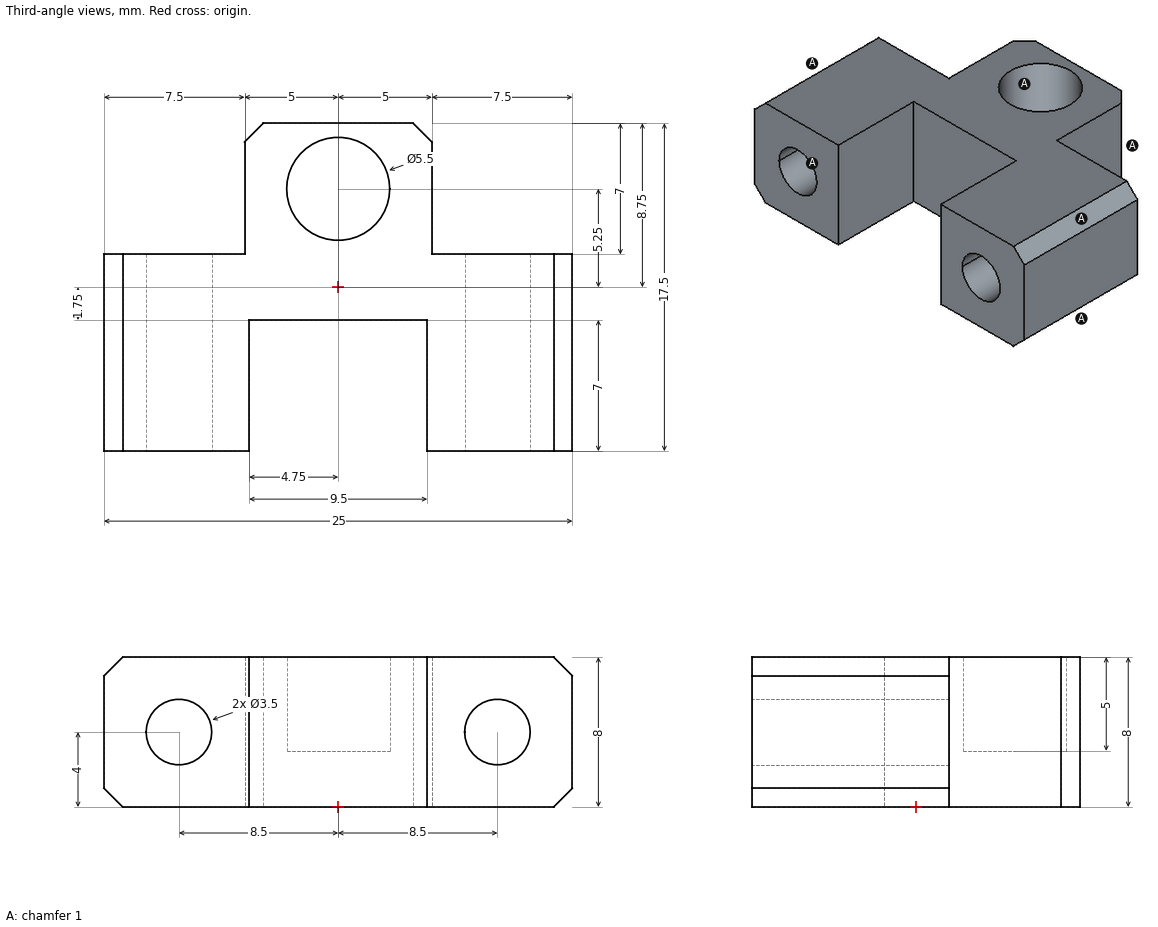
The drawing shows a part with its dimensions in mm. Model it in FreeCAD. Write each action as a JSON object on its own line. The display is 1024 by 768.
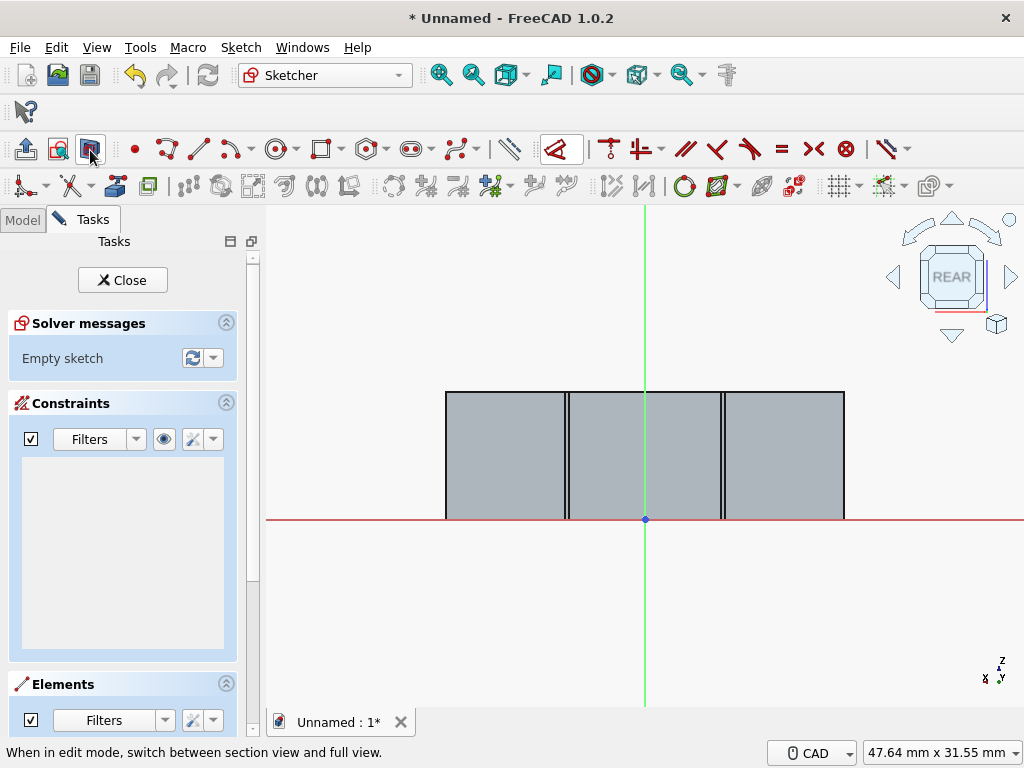
{"action": "key", "text": "g c"}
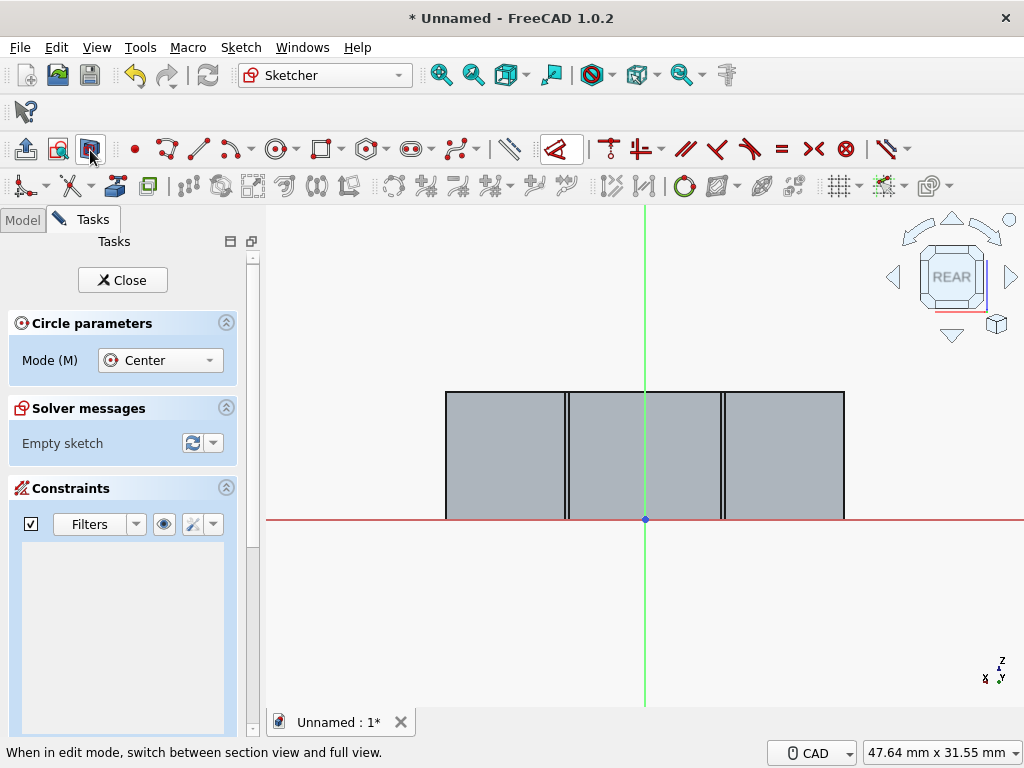
{"action": "left_click", "coordinate": [780, 456]}
{"action": "mouse_move", "coordinate": [800, 436]}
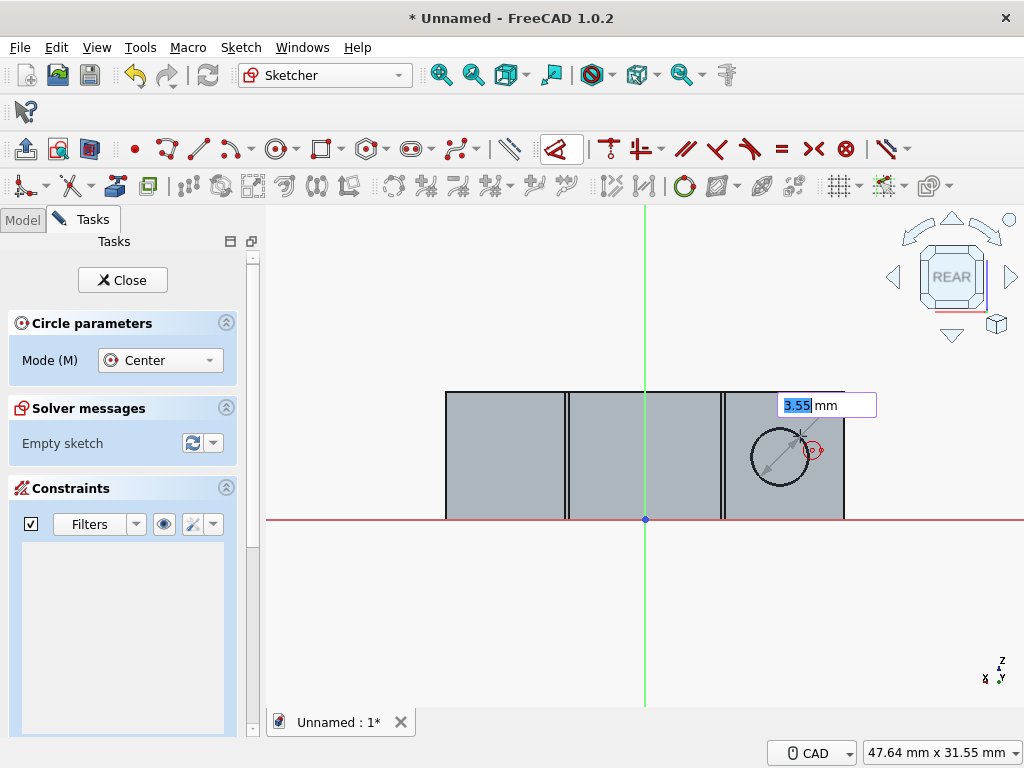
{"action": "type", "text": "3.5"}
{"action": "key", "text": "Return"}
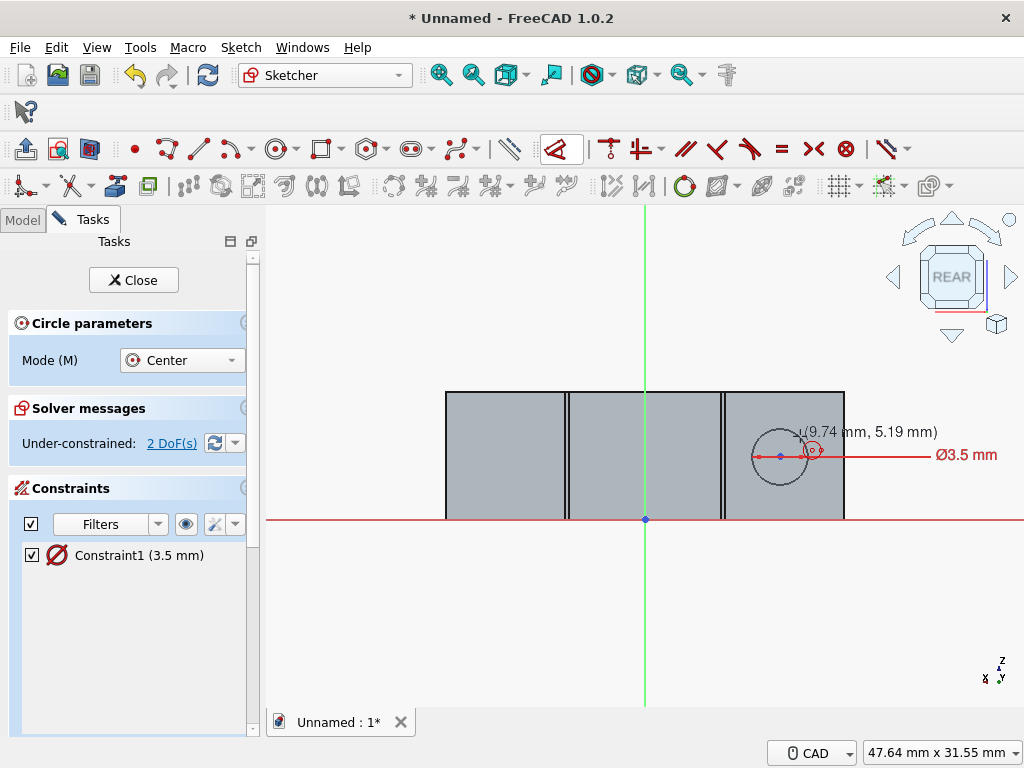
{"action": "left_click", "coordinate": [510, 456]}
{"action": "mouse_move", "coordinate": [529, 436]}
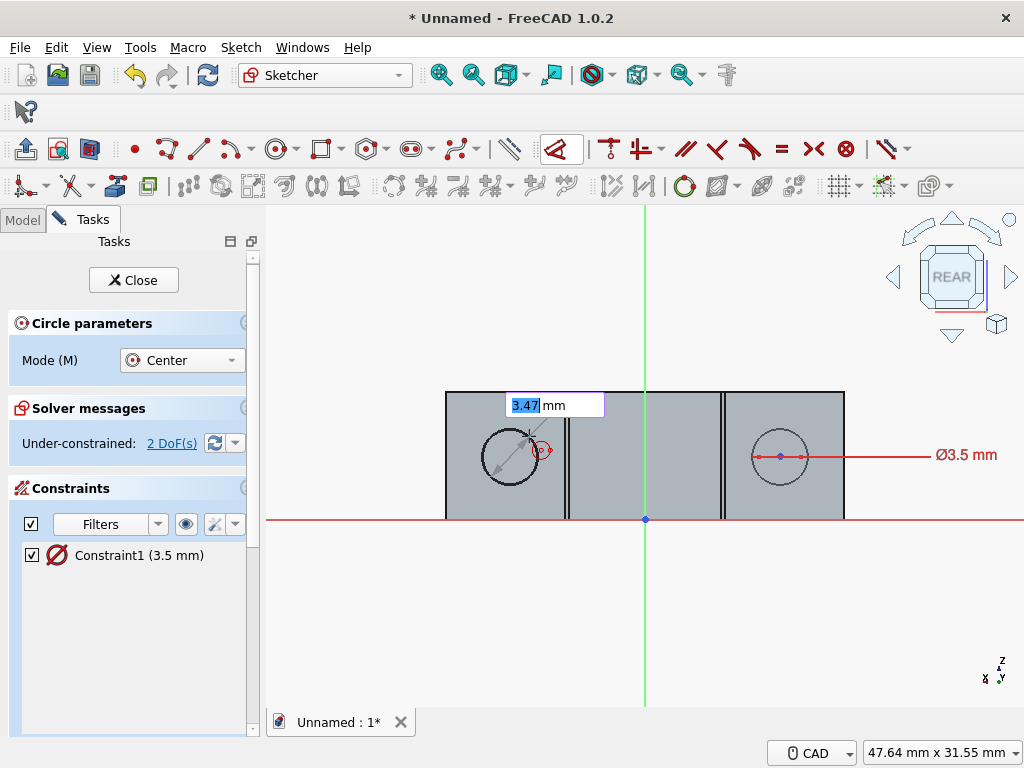
{"action": "type", "text": "3.5"}
{"action": "key", "text": "Return"}
{"action": "key", "text": "Escape"}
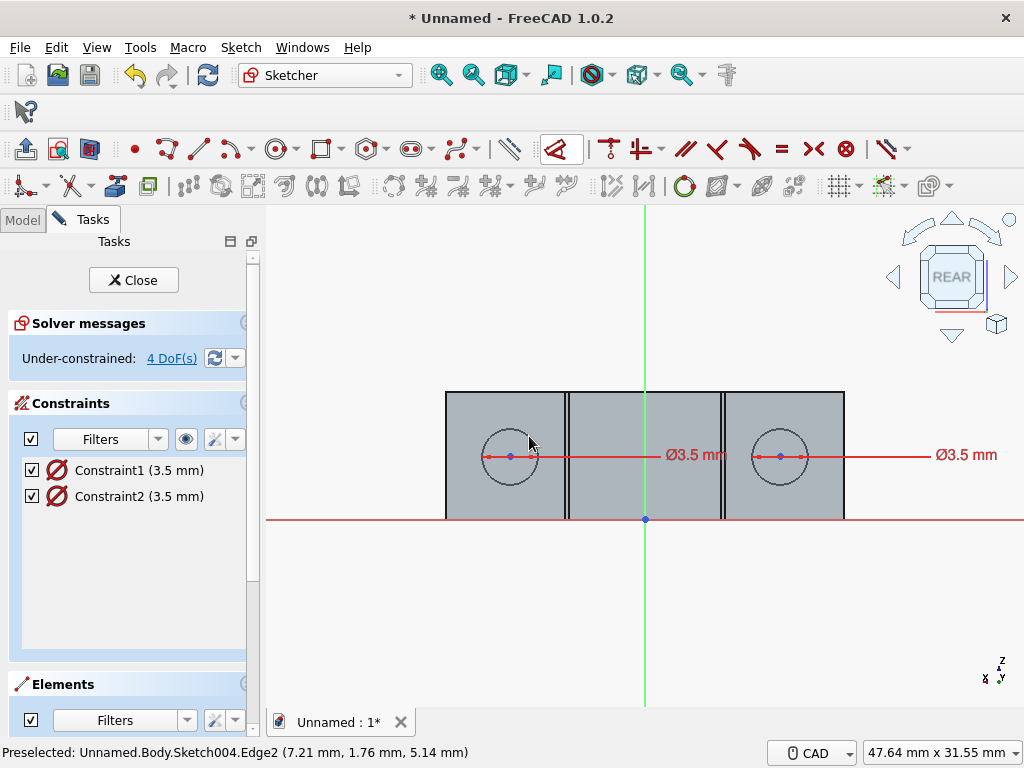
{"action": "left_click", "coordinate": [780, 457]}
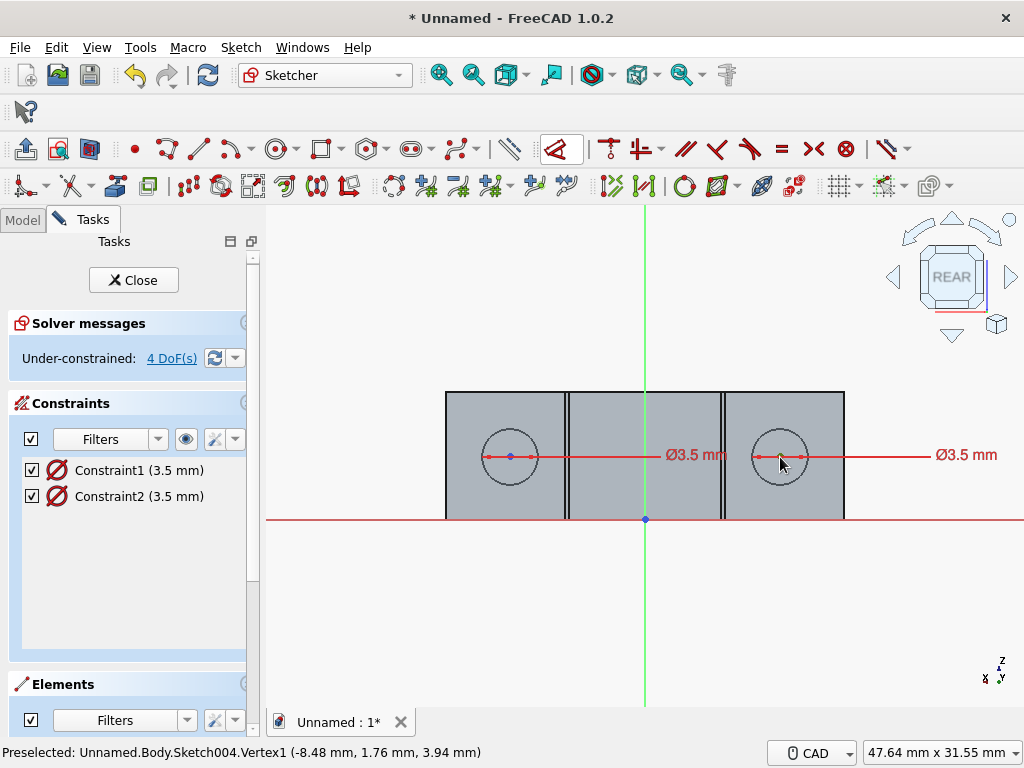
{"action": "key", "text": "i"}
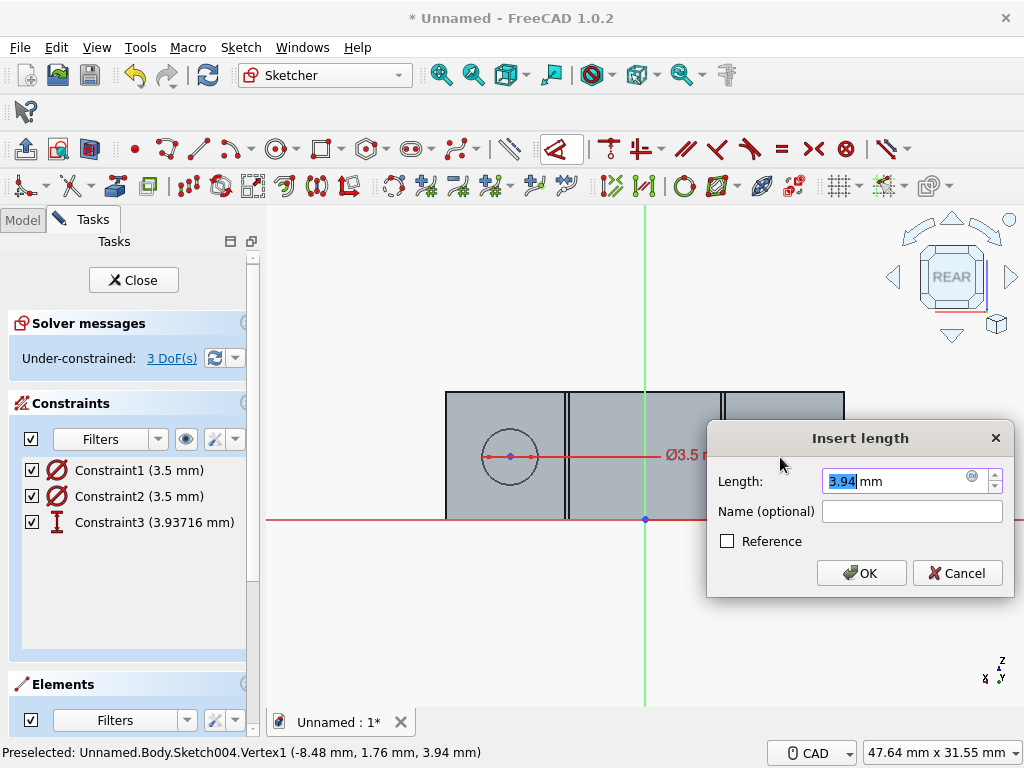
{"action": "type", "text": "4"}
{"action": "key", "text": "Return"}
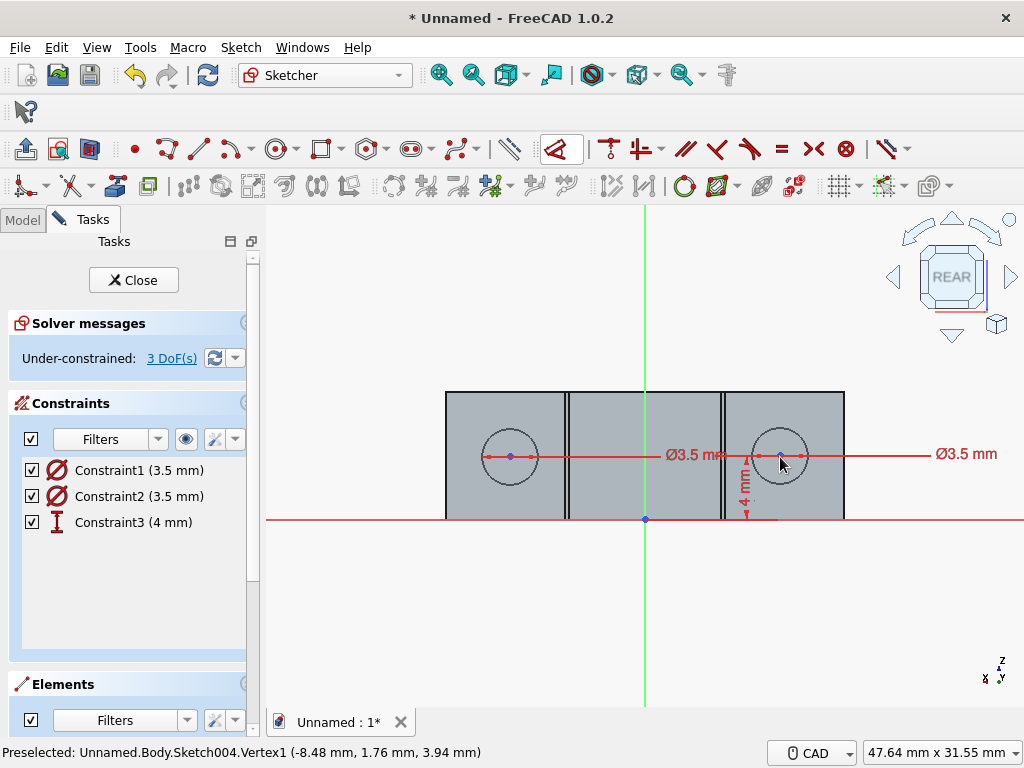
{"action": "left_click", "coordinate": [510, 457]}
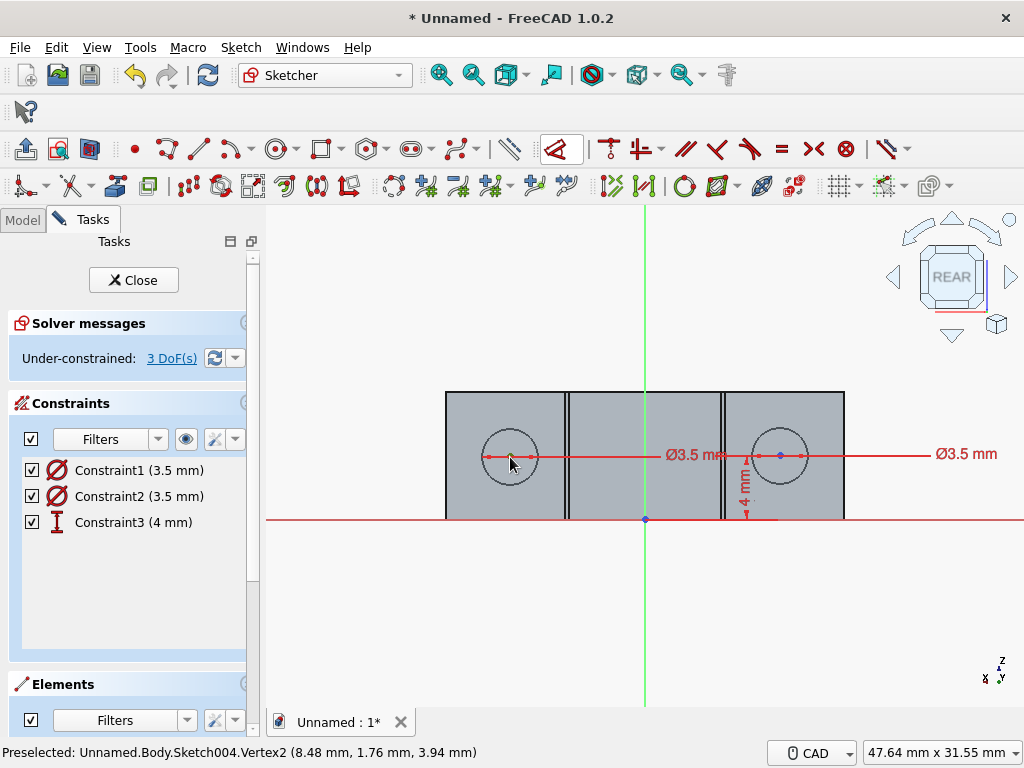
{"action": "key", "text": "i"}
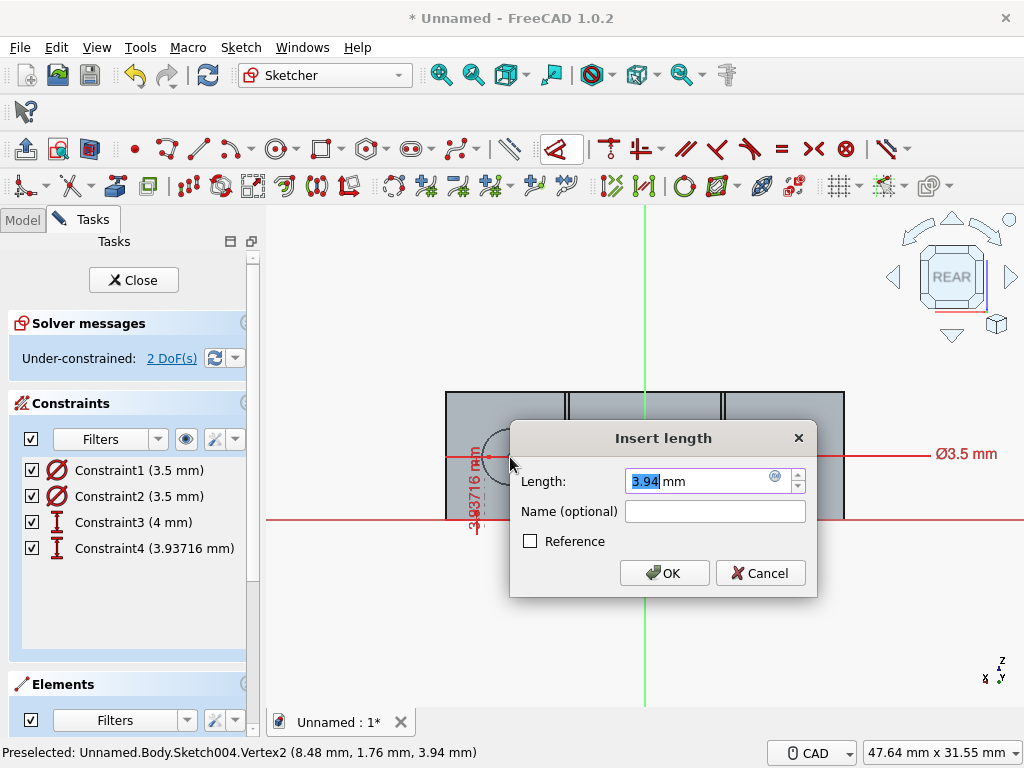
{"action": "type", "text": "4"}
{"action": "key", "text": "Return"}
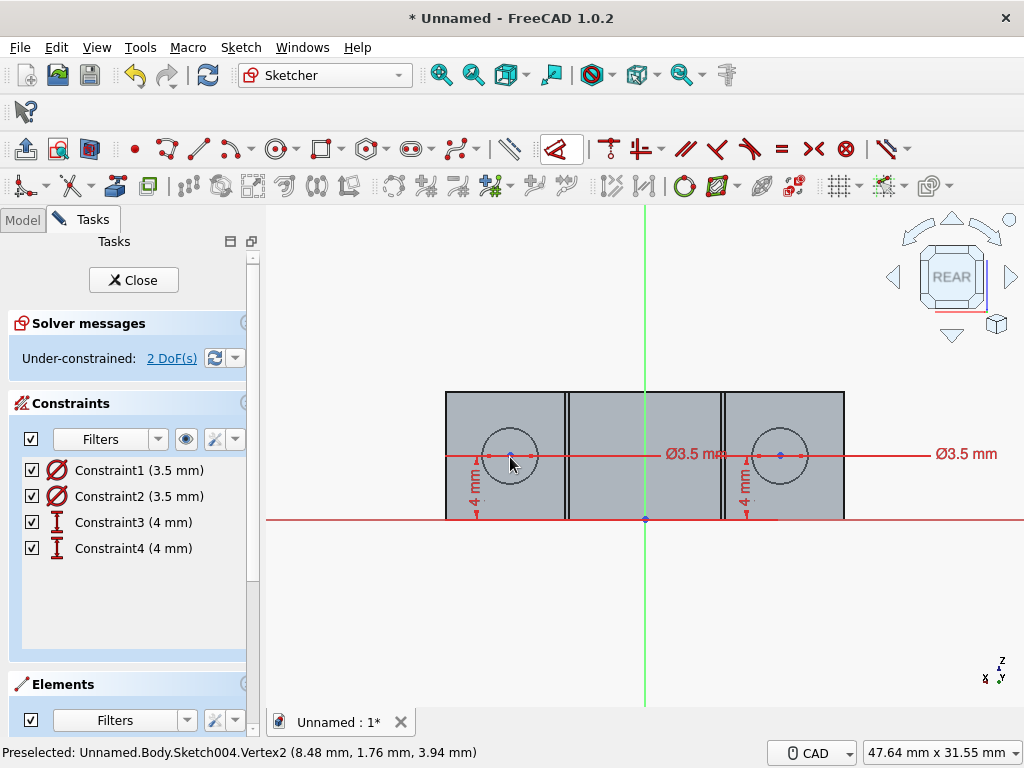
{"action": "left_click", "coordinate": [780, 456]}